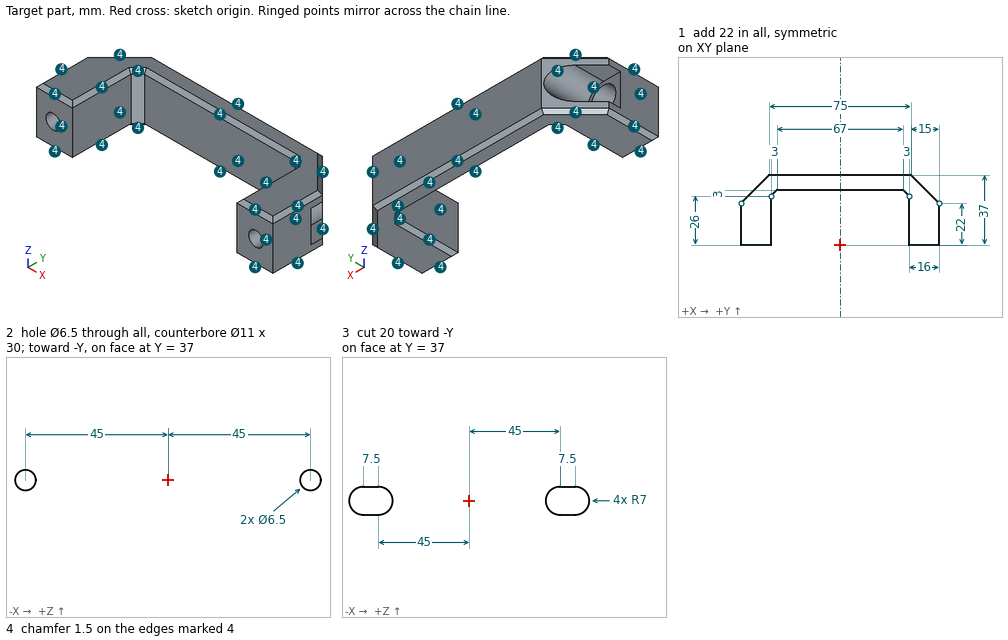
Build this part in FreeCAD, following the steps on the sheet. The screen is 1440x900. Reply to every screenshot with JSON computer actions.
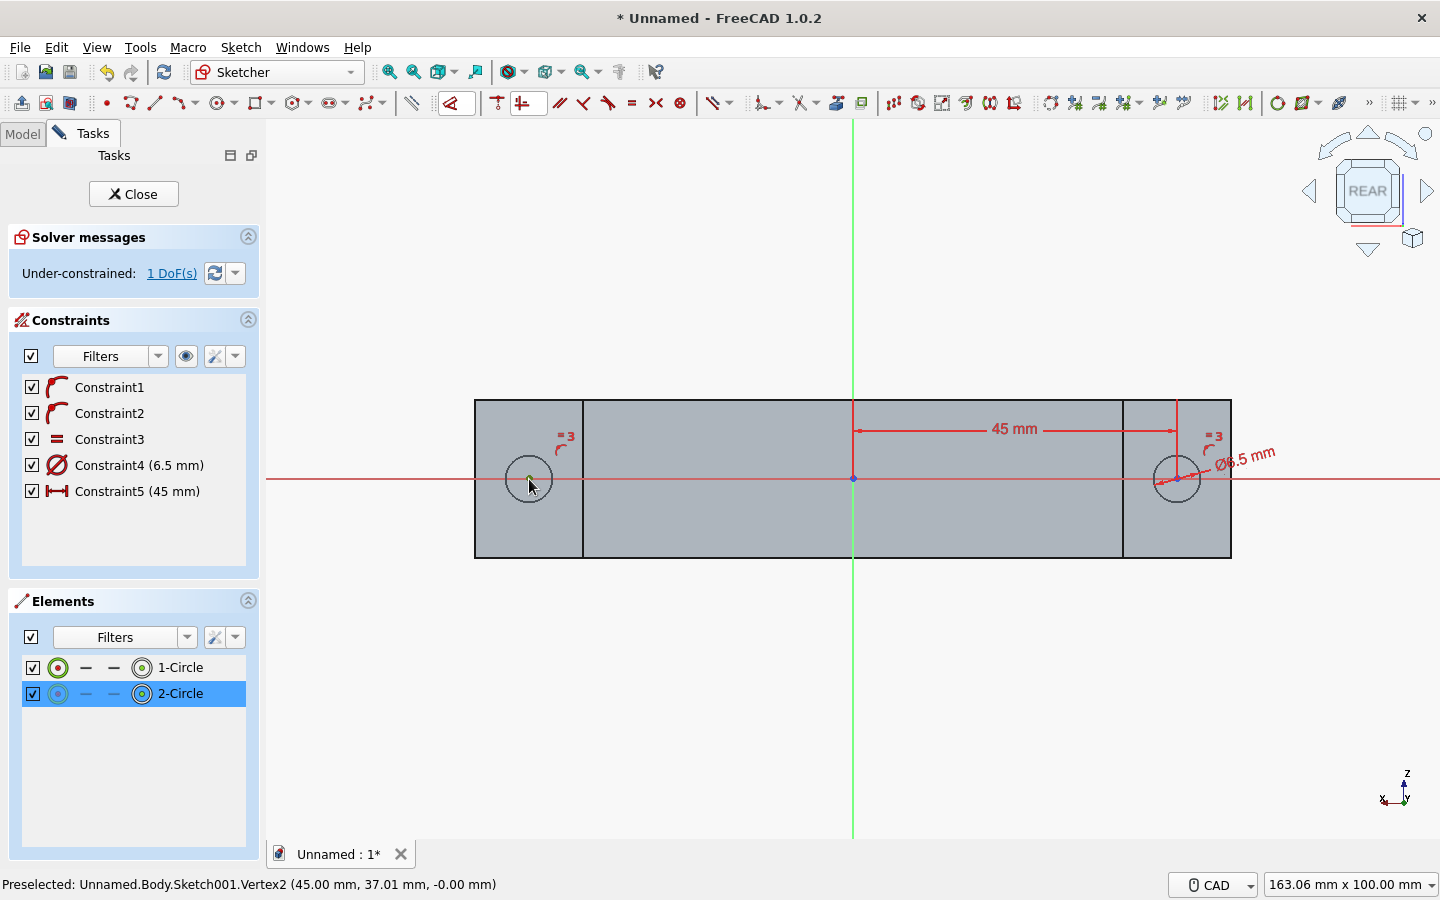
{"action": "left_click", "coordinate": [470, 104]}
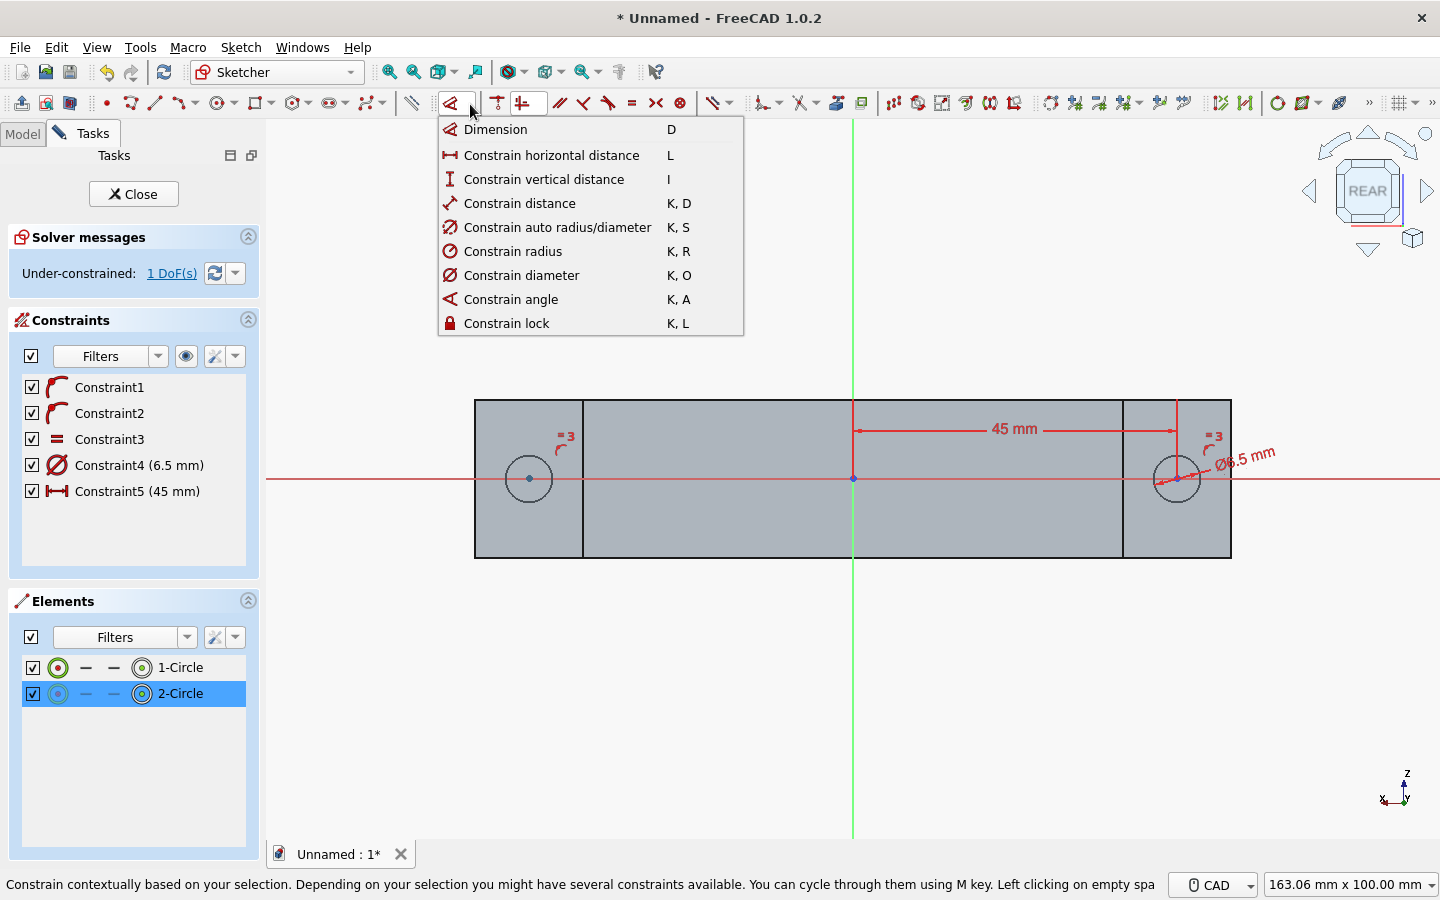
{"action": "left_click", "coordinate": [591, 155]}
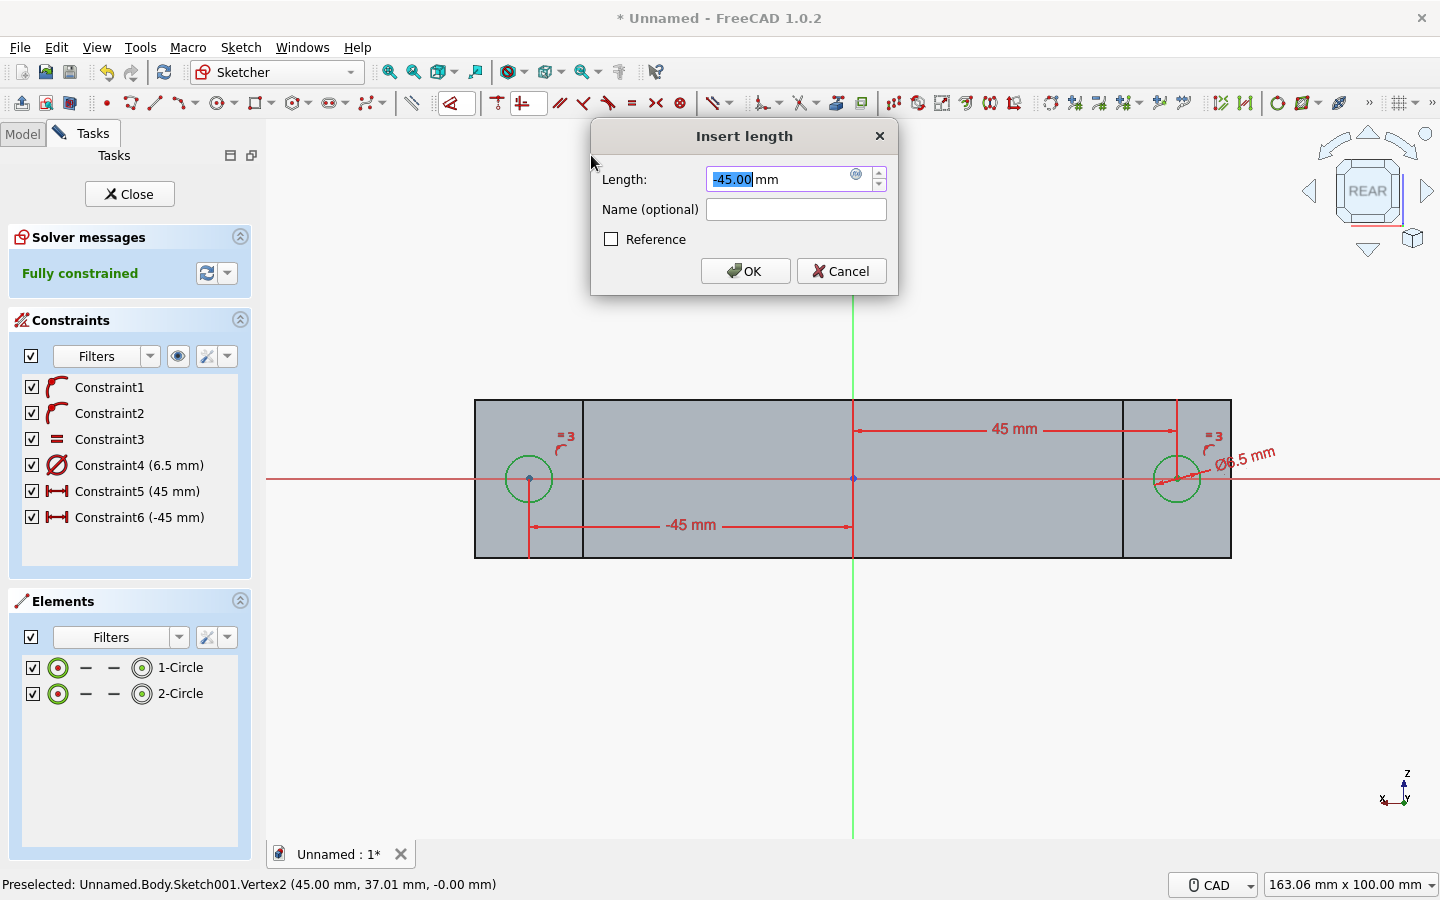
{"action": "type", "text": "-45"}
{"action": "key", "text": "Return"}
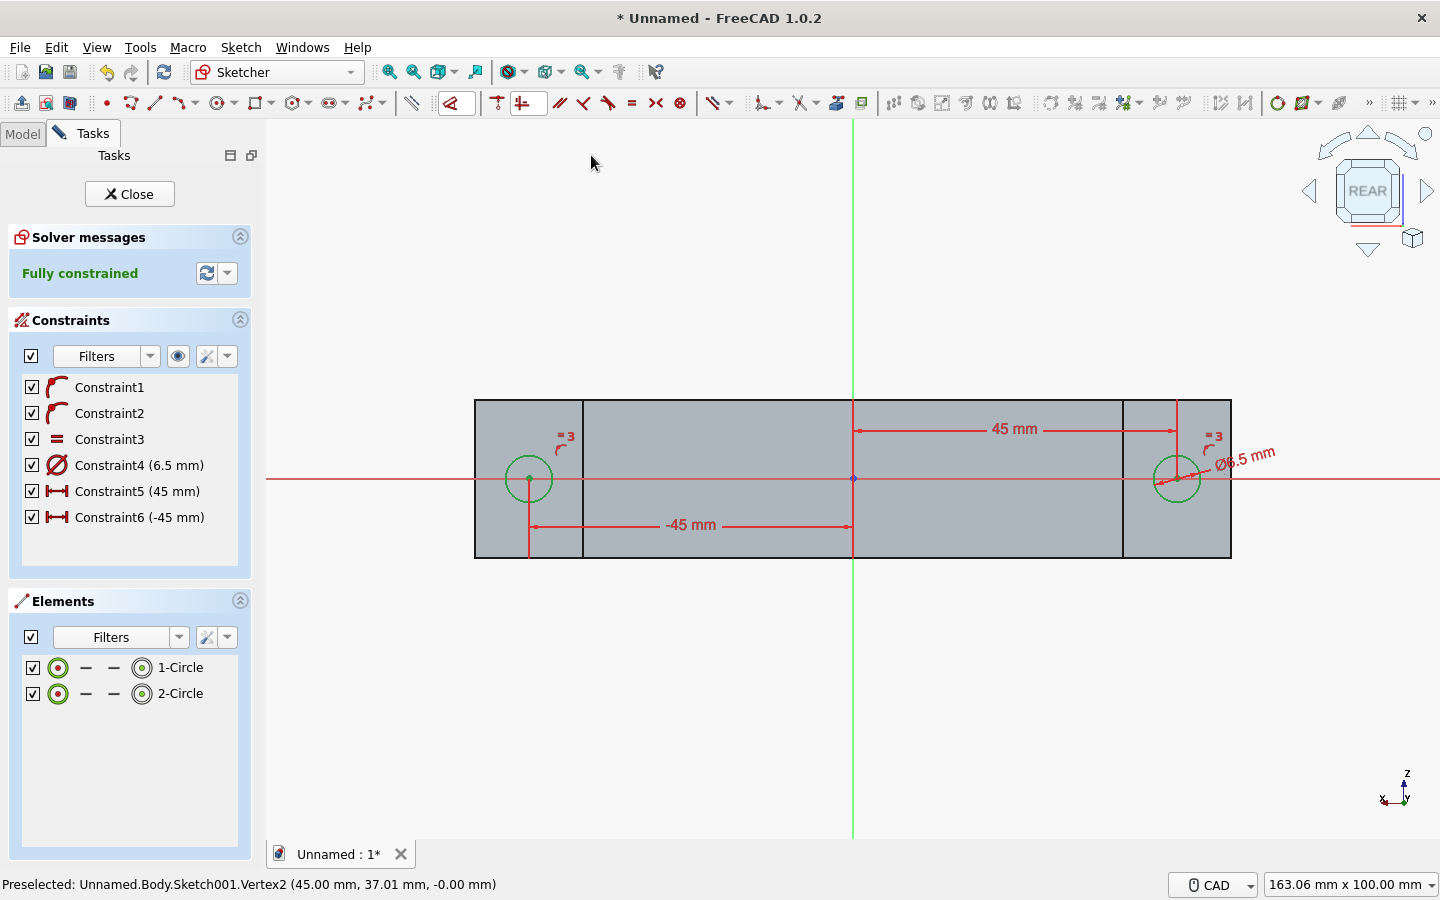
{"action": "left_click", "coordinate": [130, 194]}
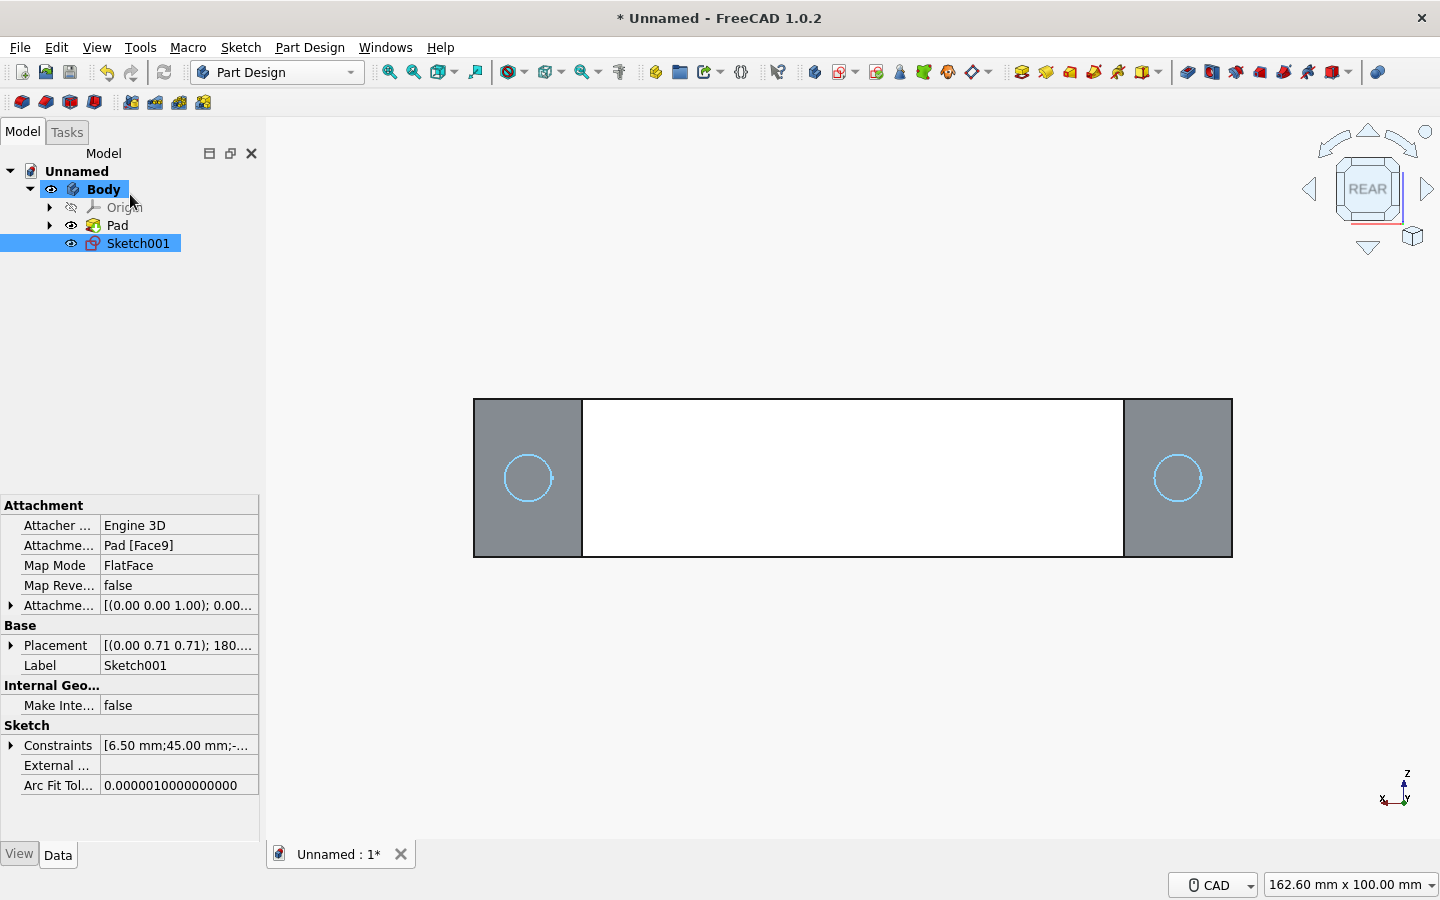
{"action": "left_click", "coordinate": [1212, 72]}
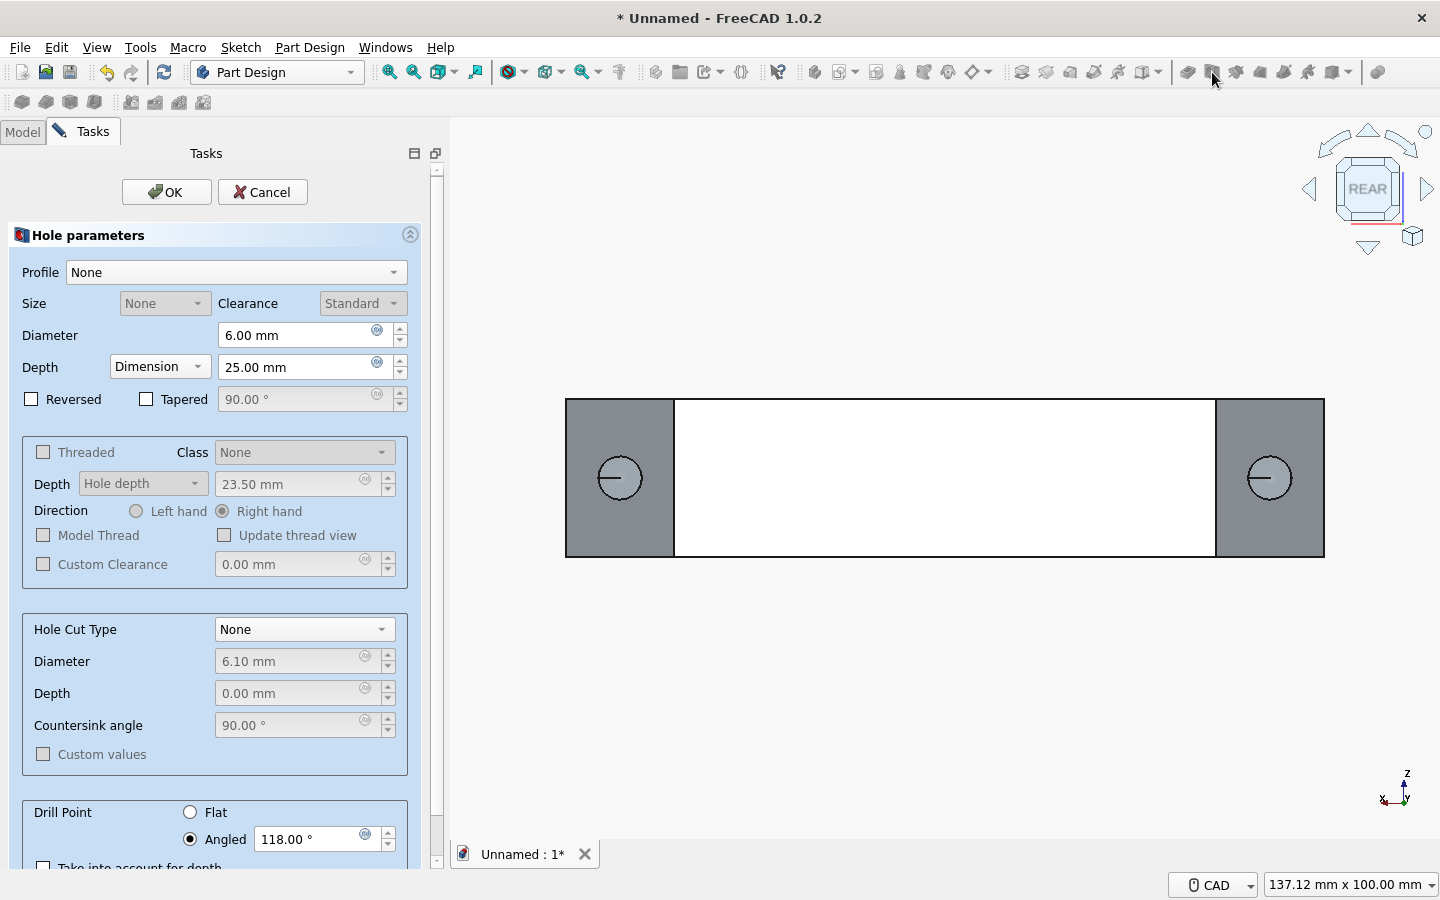
{"action": "triple_click", "coordinate": [305, 335]}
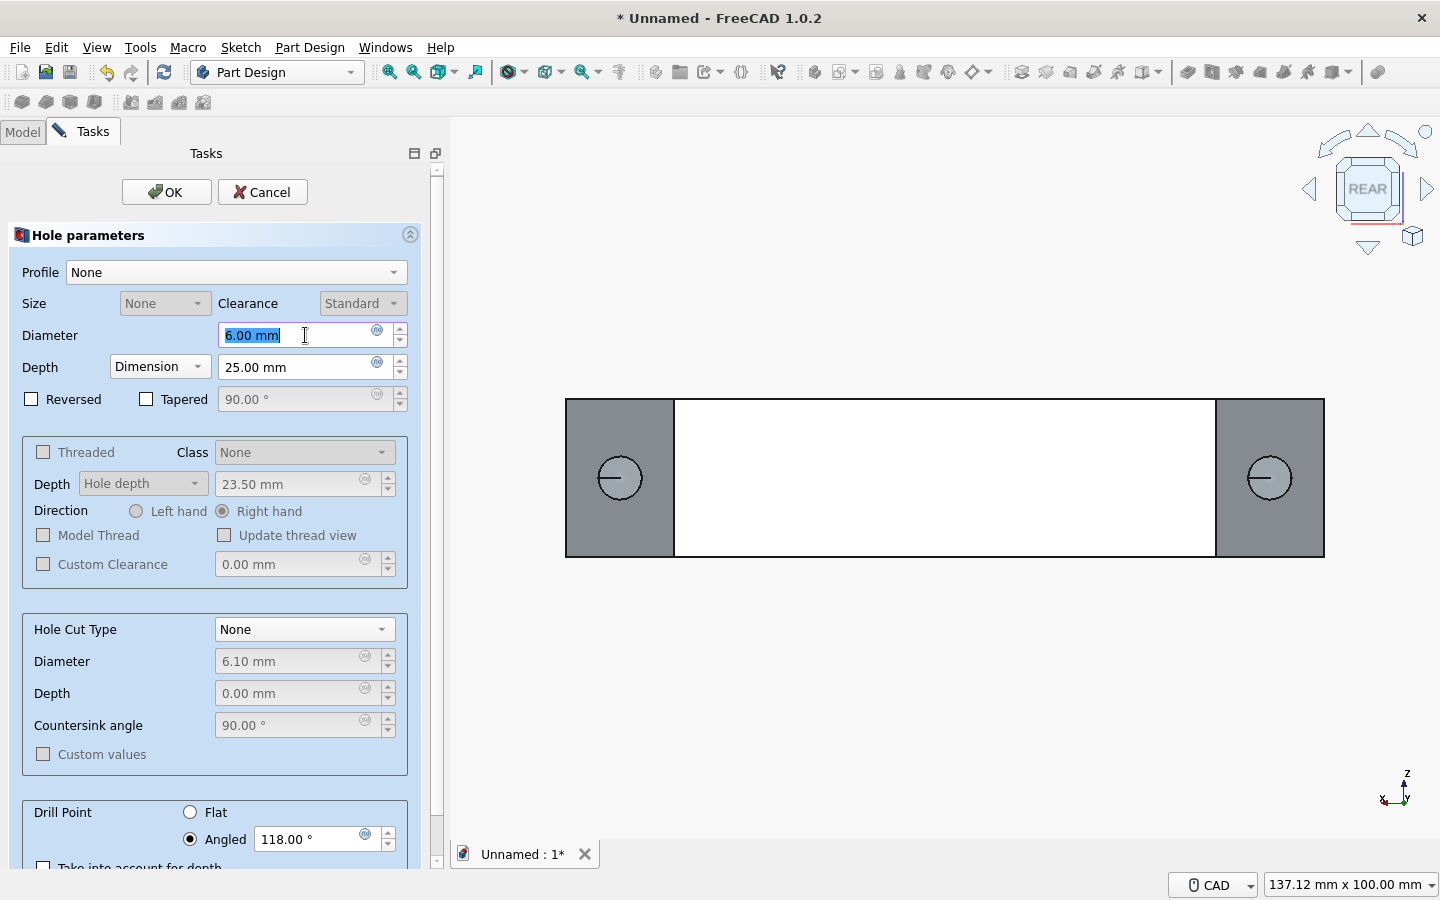
{"action": "type", "text": "6.5"}
{"action": "key", "text": "Tab"}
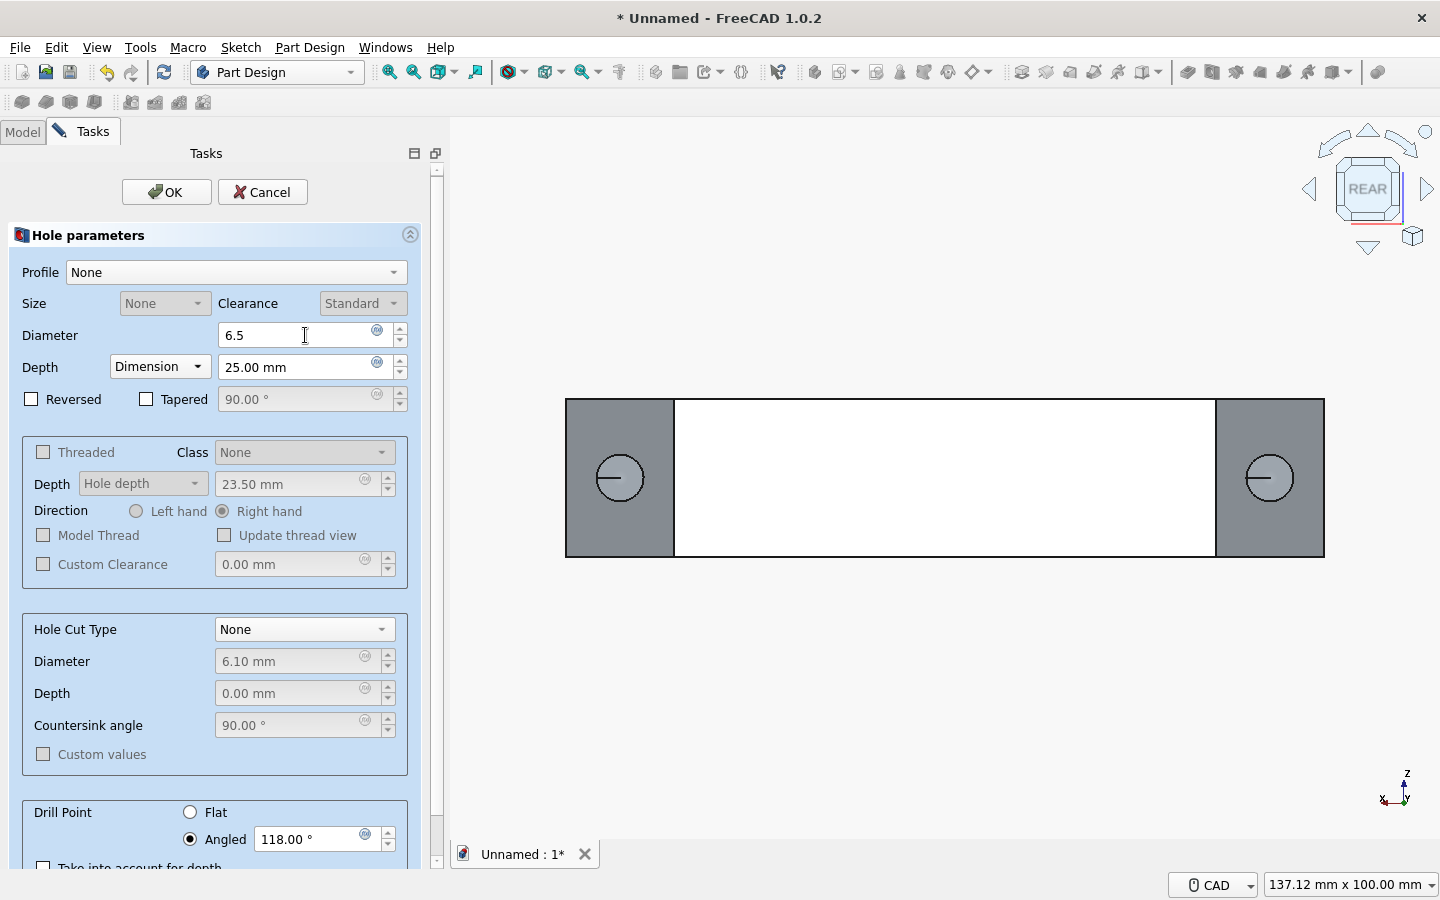
{"action": "left_click", "coordinate": [161, 366]}